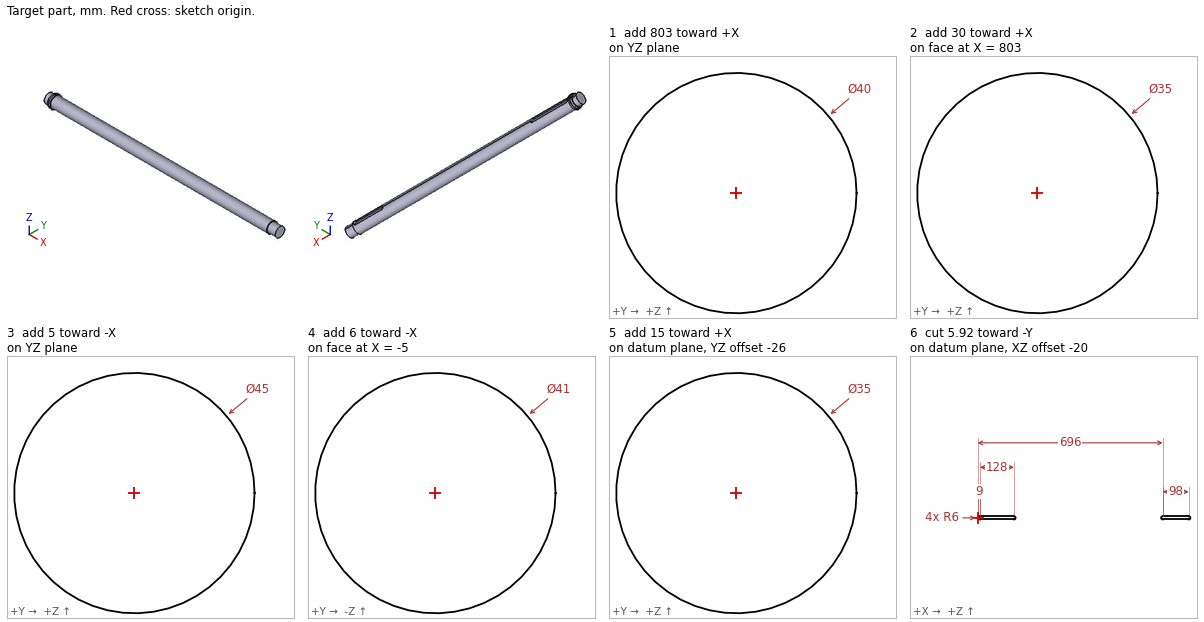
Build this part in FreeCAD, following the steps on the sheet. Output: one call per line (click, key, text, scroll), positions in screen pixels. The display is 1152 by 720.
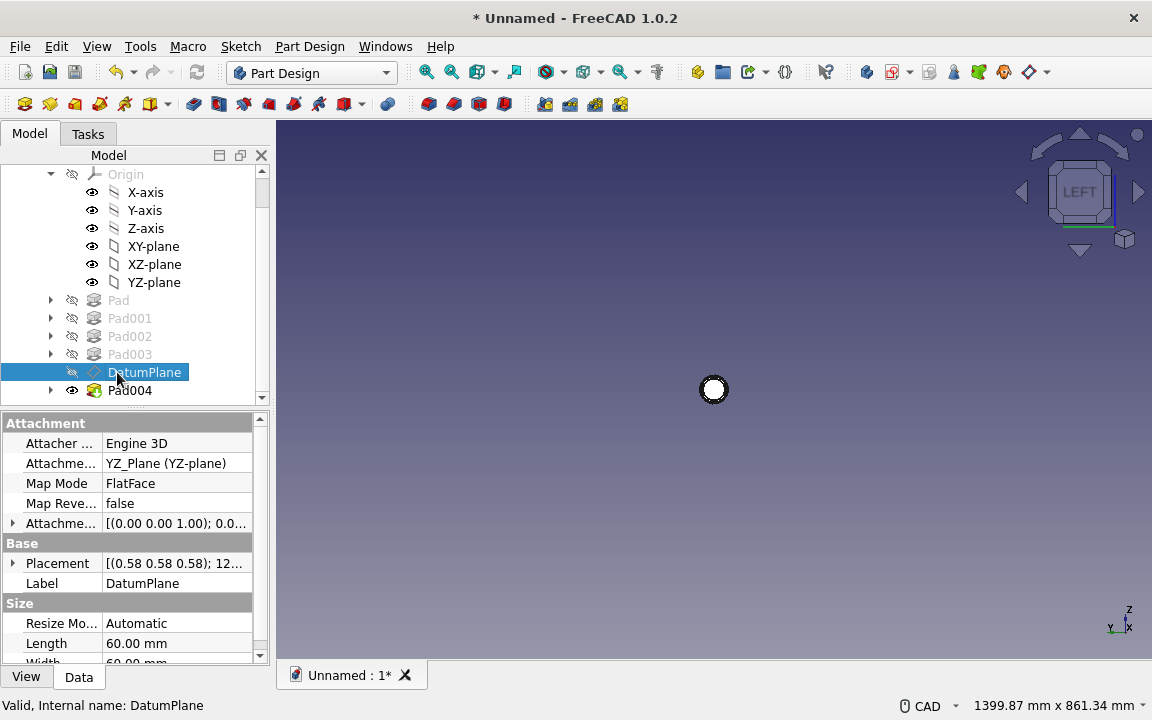
click(137, 264)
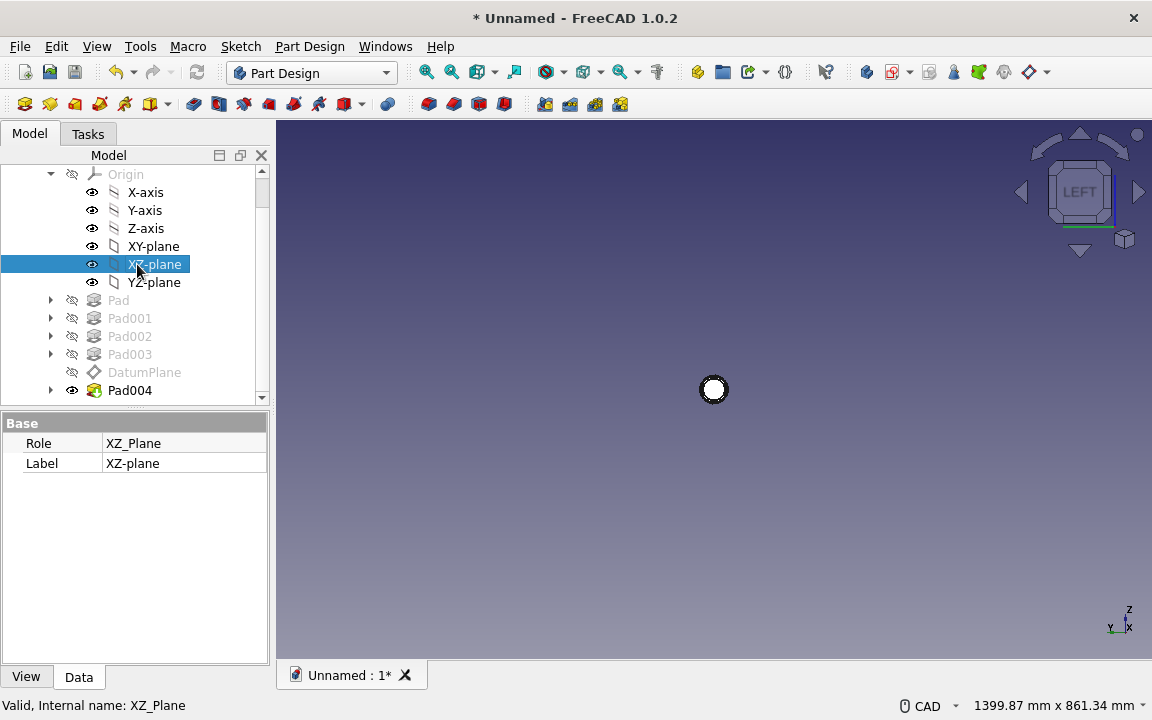
click(1028, 72)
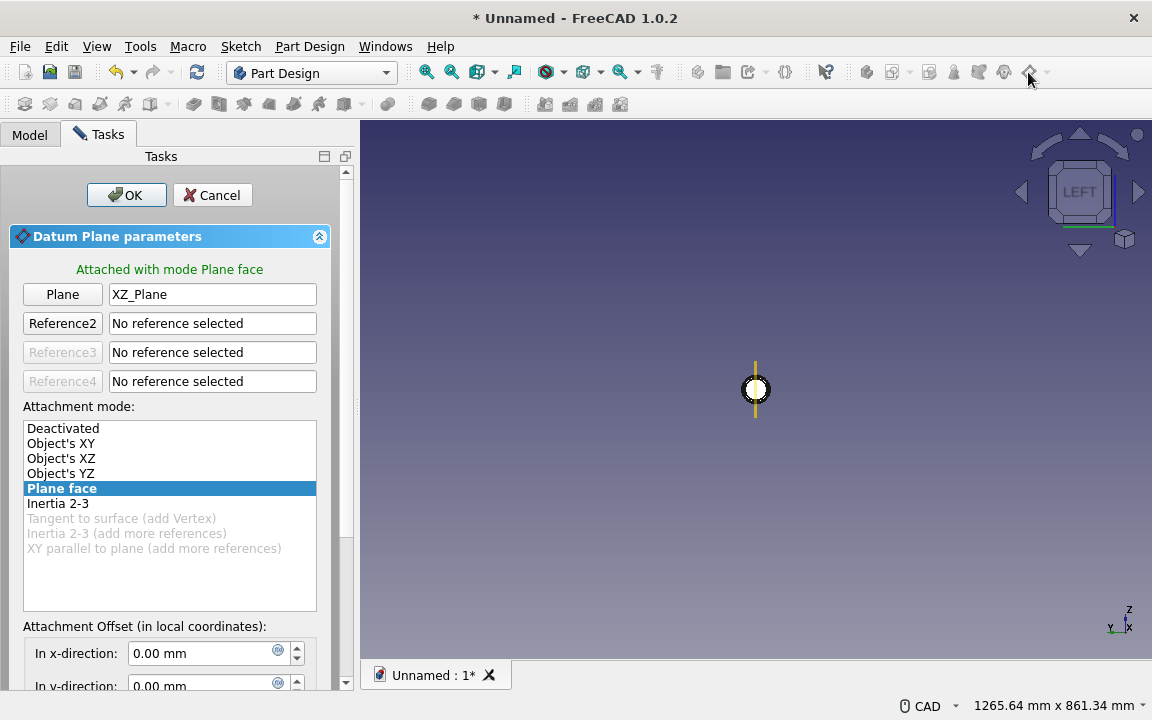
scroll(346, 428, down, 2)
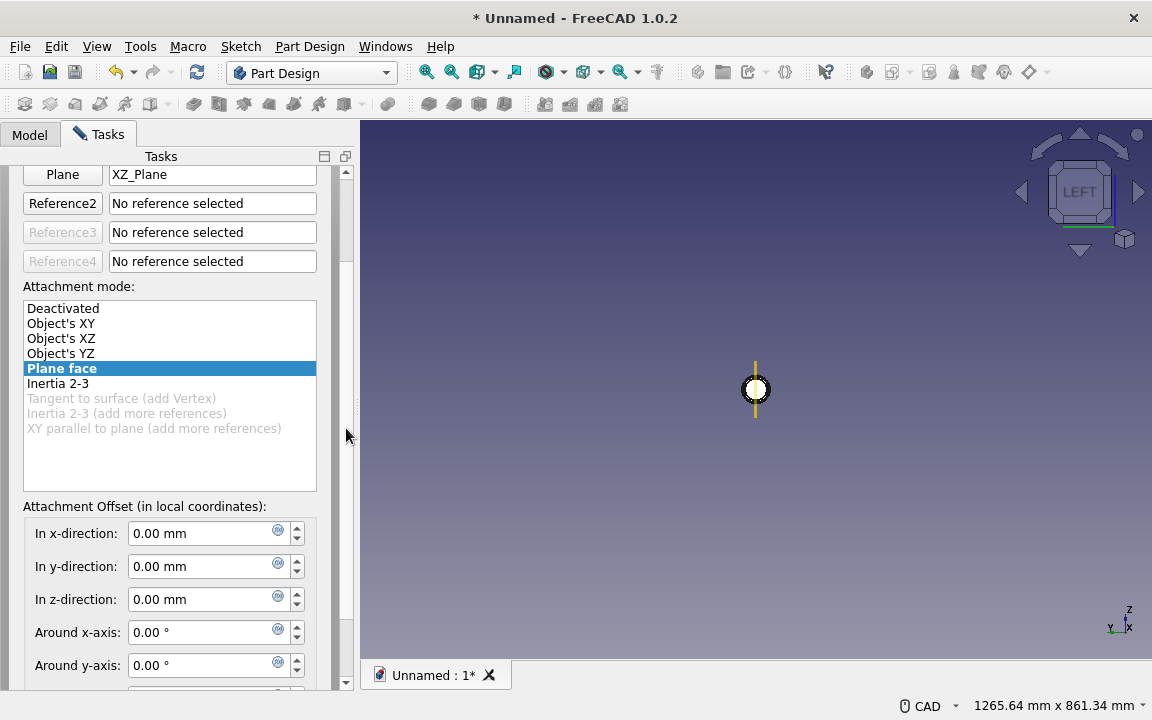
triple_click(210, 600)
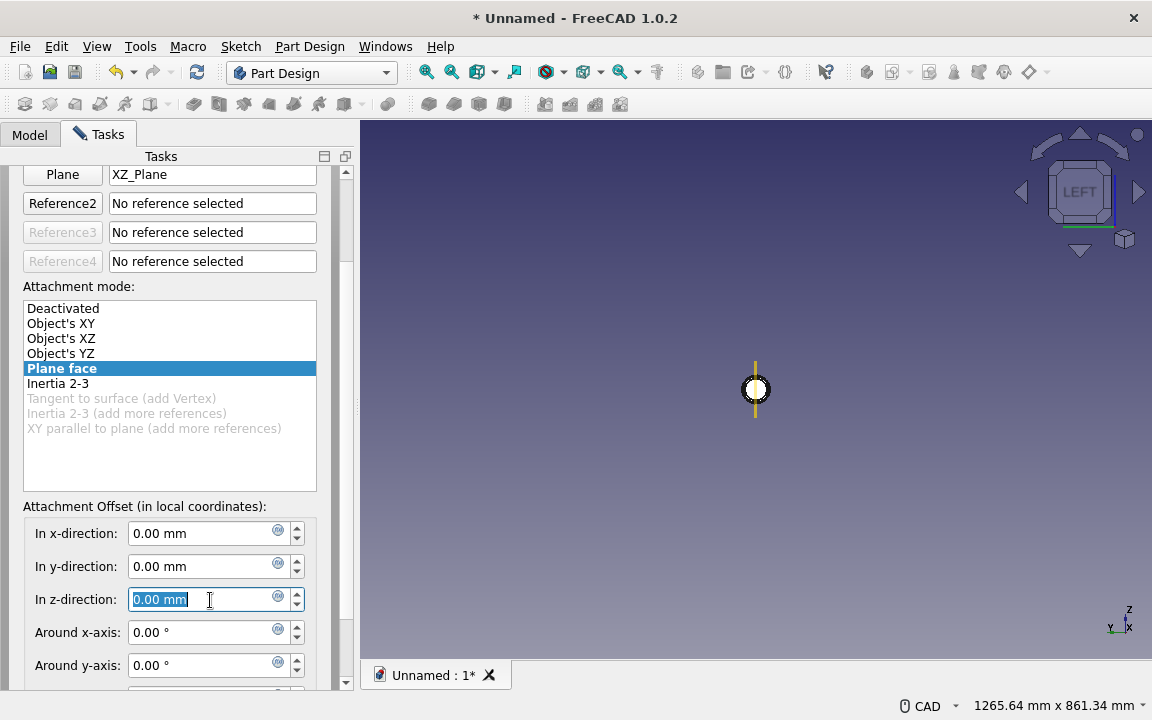
text(-20)
key(Tab)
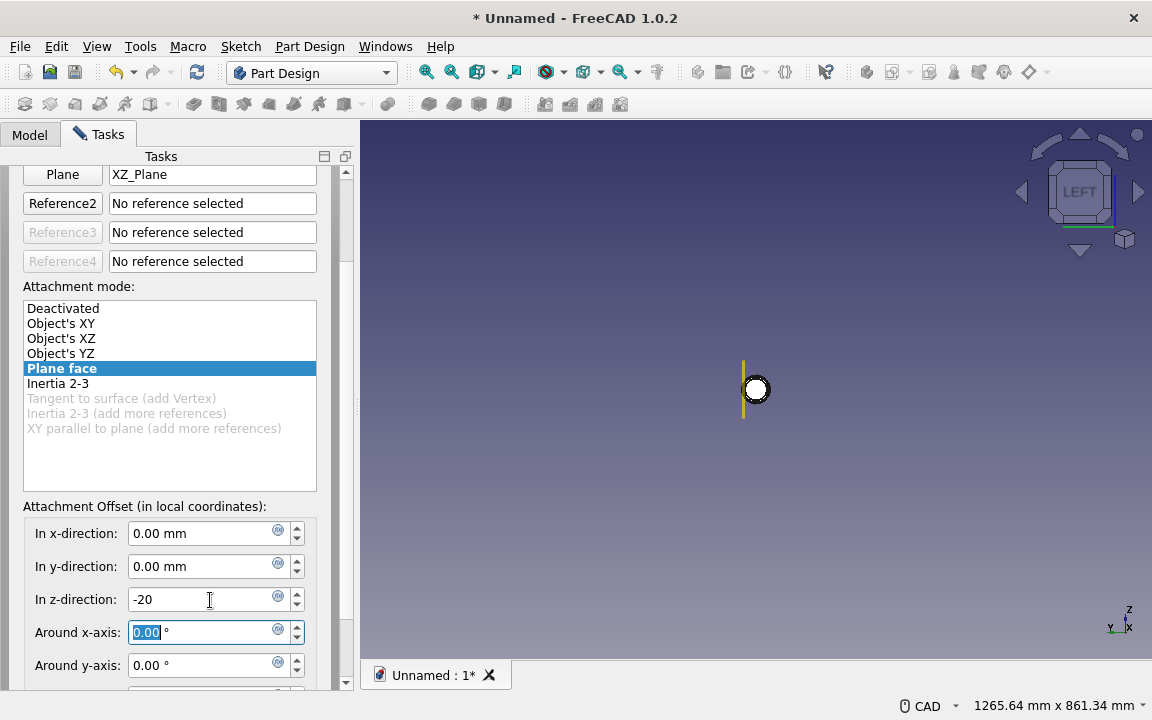
scroll(346, 428, up, 3)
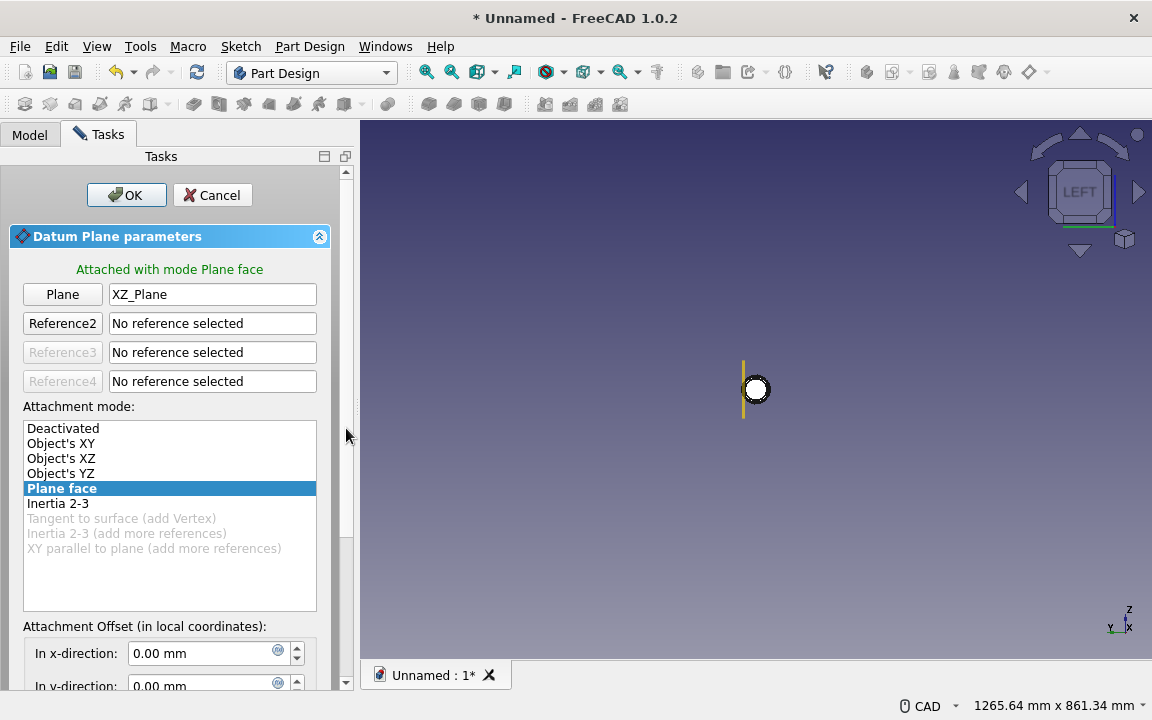
click(127, 195)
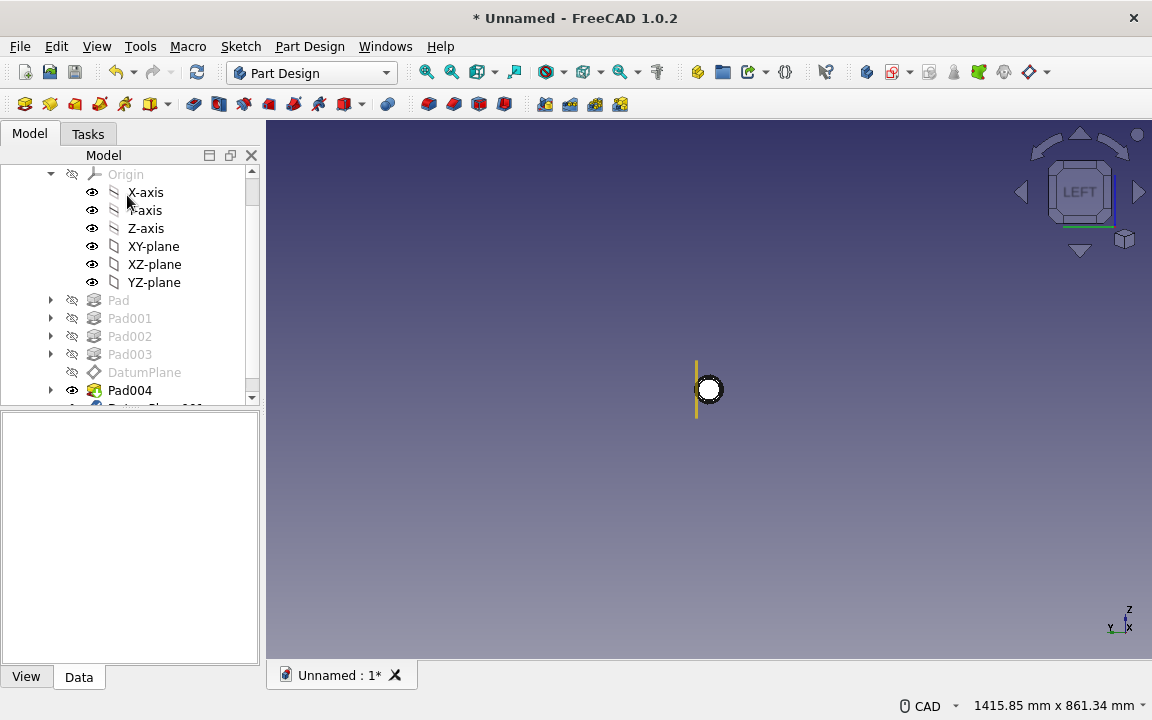
scroll(141, 278, down, 3)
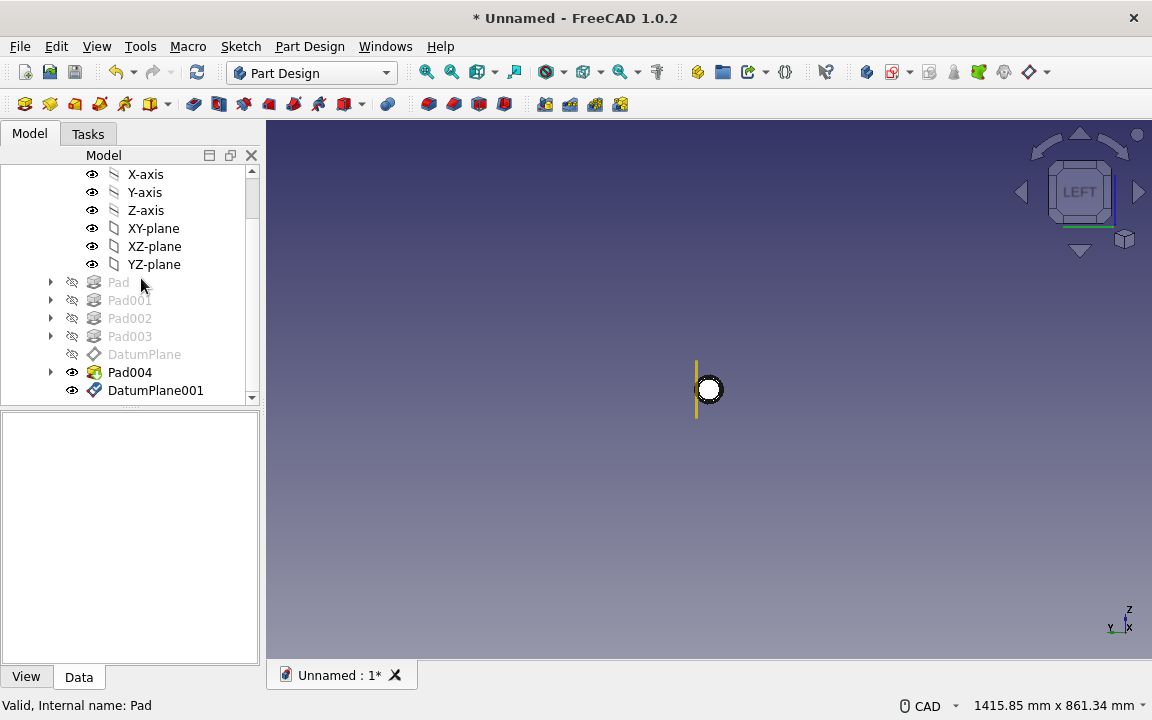
click(117, 390)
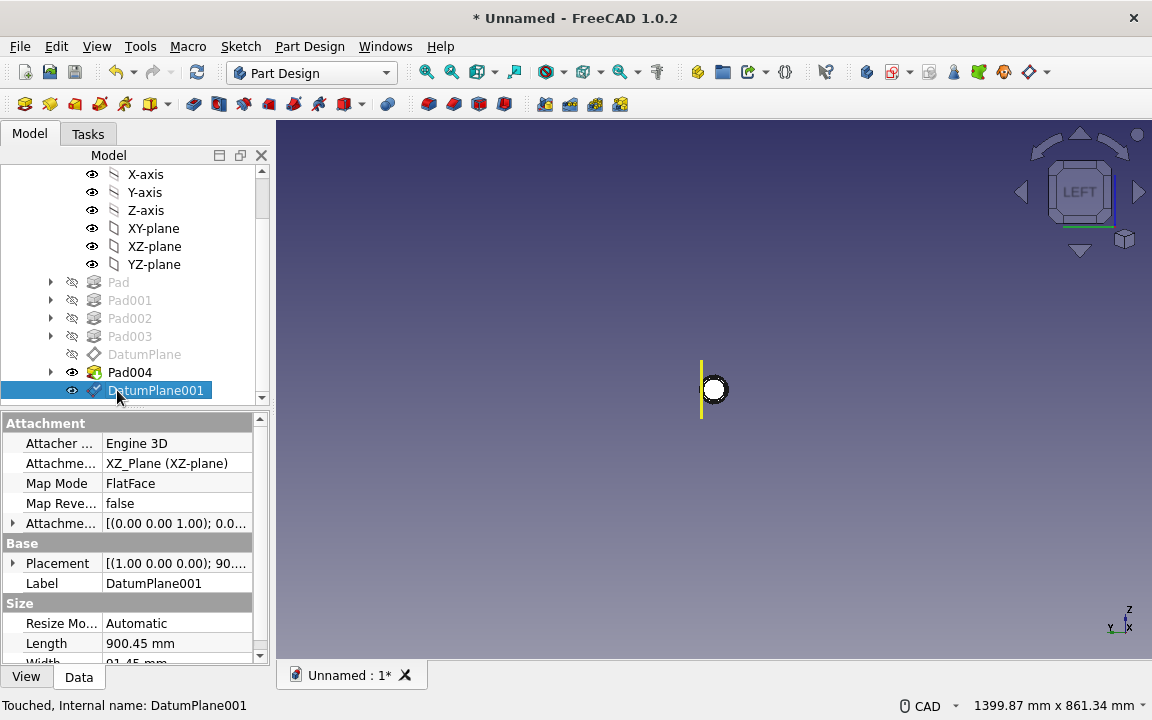
click(892, 72)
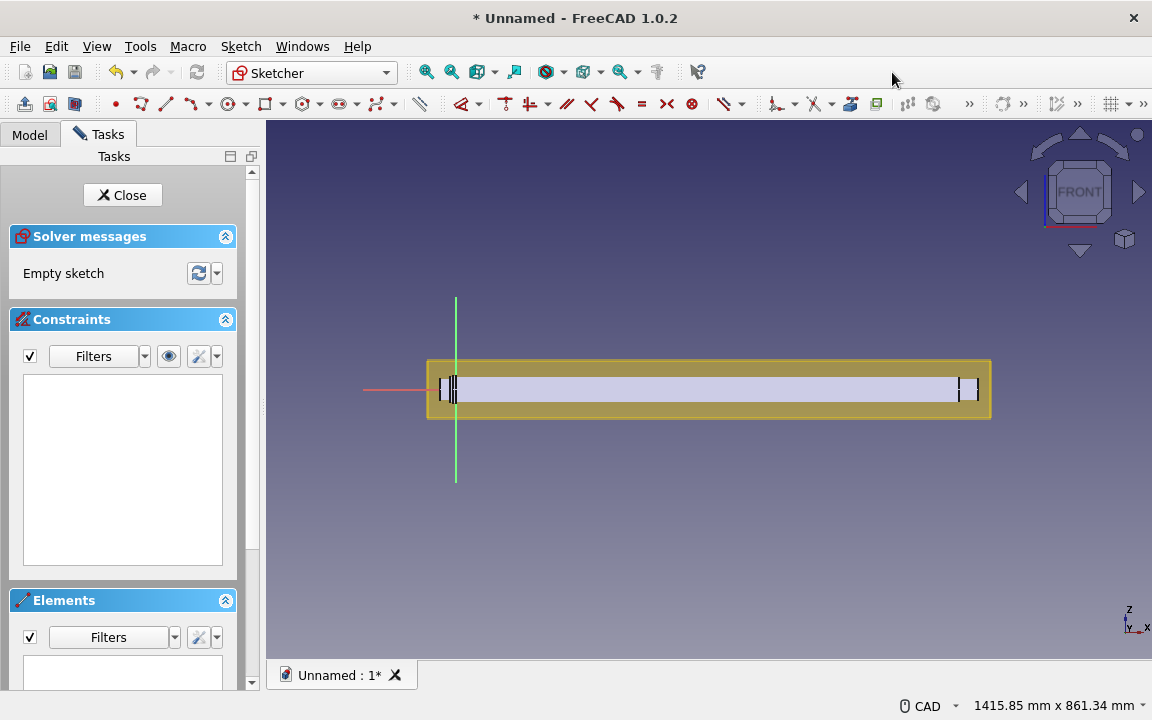
click(75, 104)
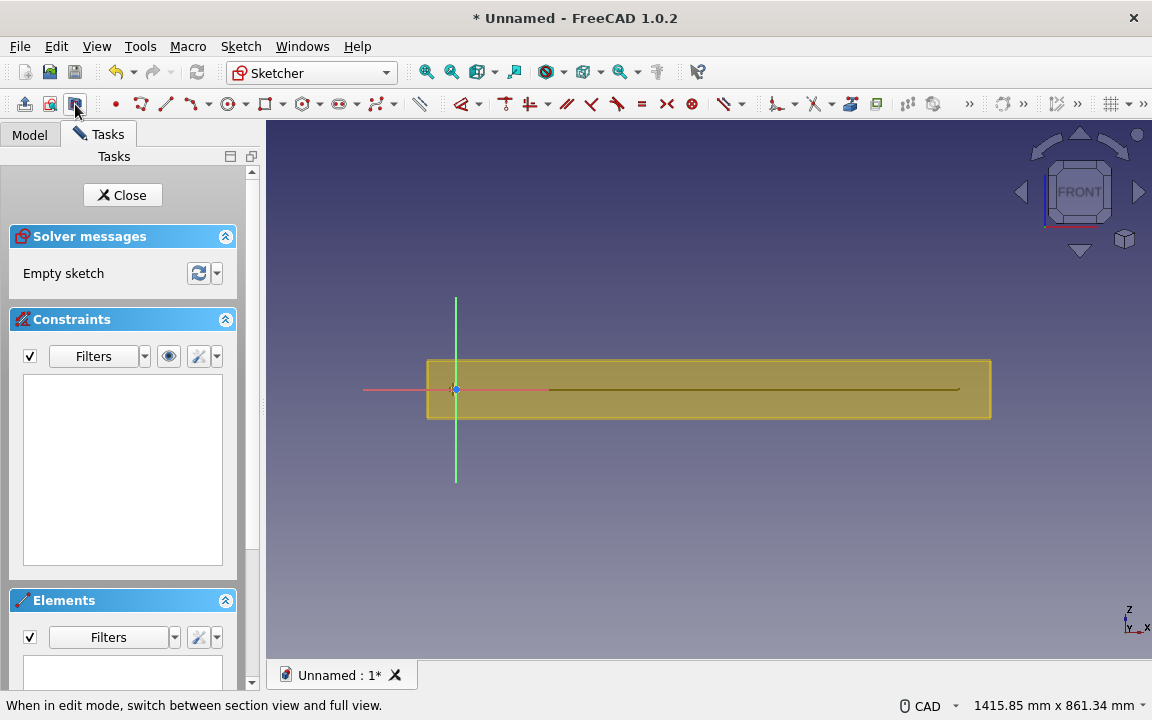
click(338, 104)